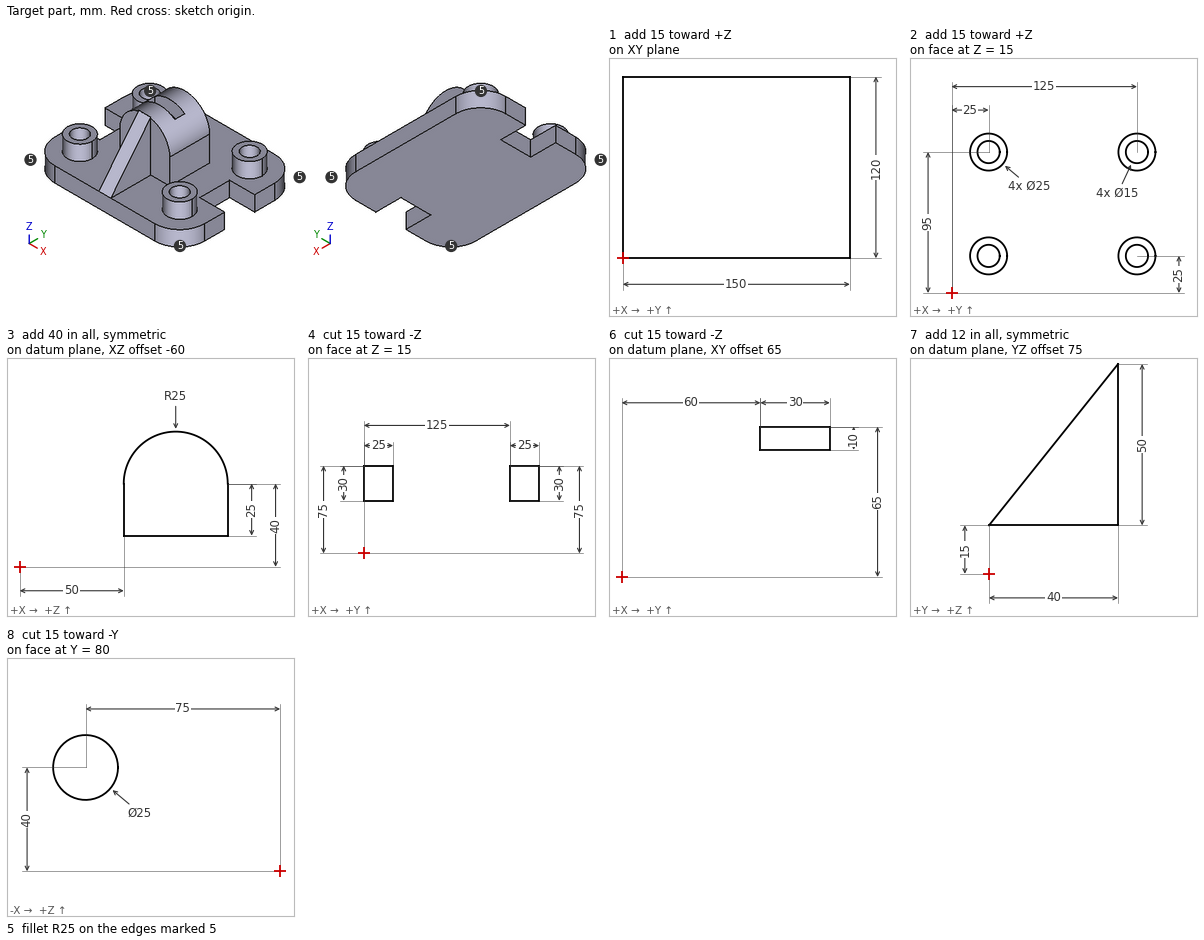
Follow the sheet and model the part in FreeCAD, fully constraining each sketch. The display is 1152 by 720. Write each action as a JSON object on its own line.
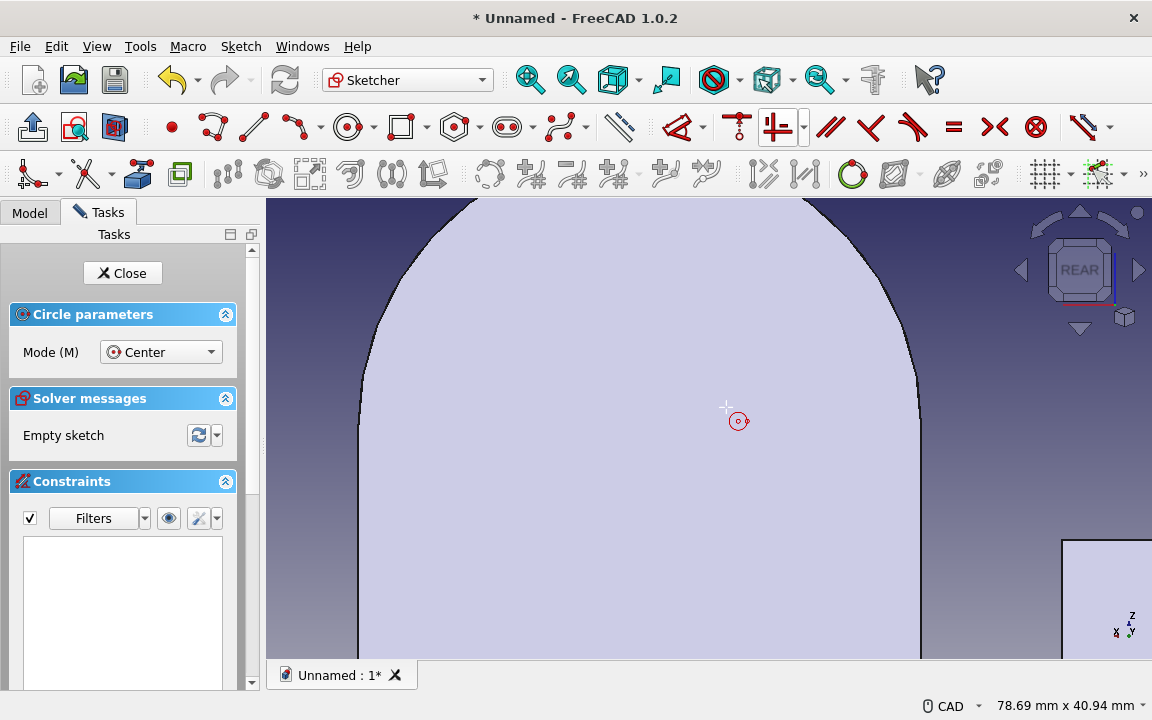
{"action": "left_click", "coordinate": [640, 427]}
{"action": "left_click", "coordinate": [739, 328]}
{"action": "key", "text": "Escape"}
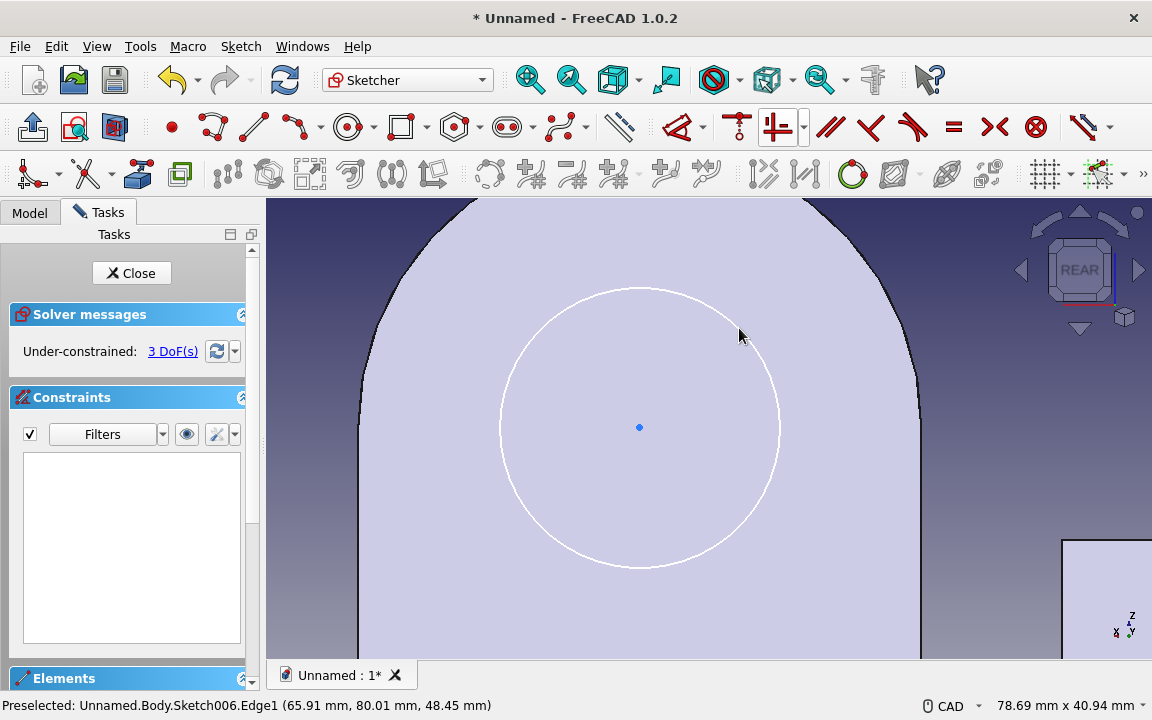
{"action": "left_click", "coordinate": [676, 128]}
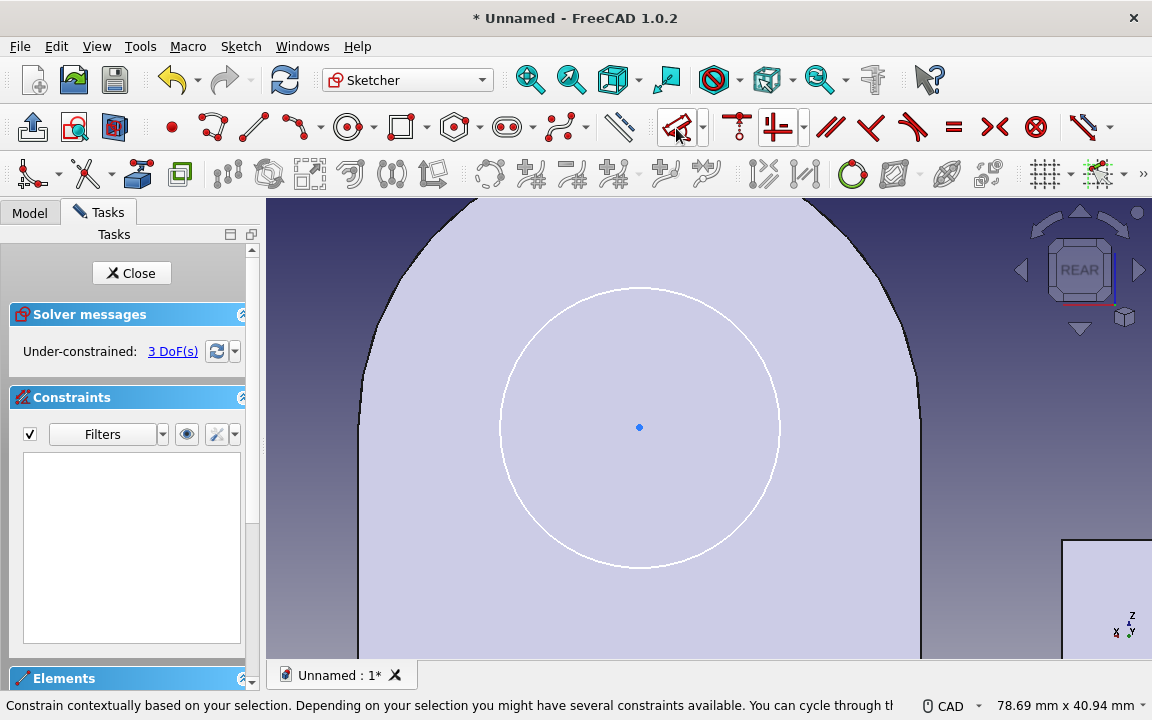
{"action": "left_click", "coordinate": [739, 329]}
{"action": "left_click", "coordinate": [762, 306]}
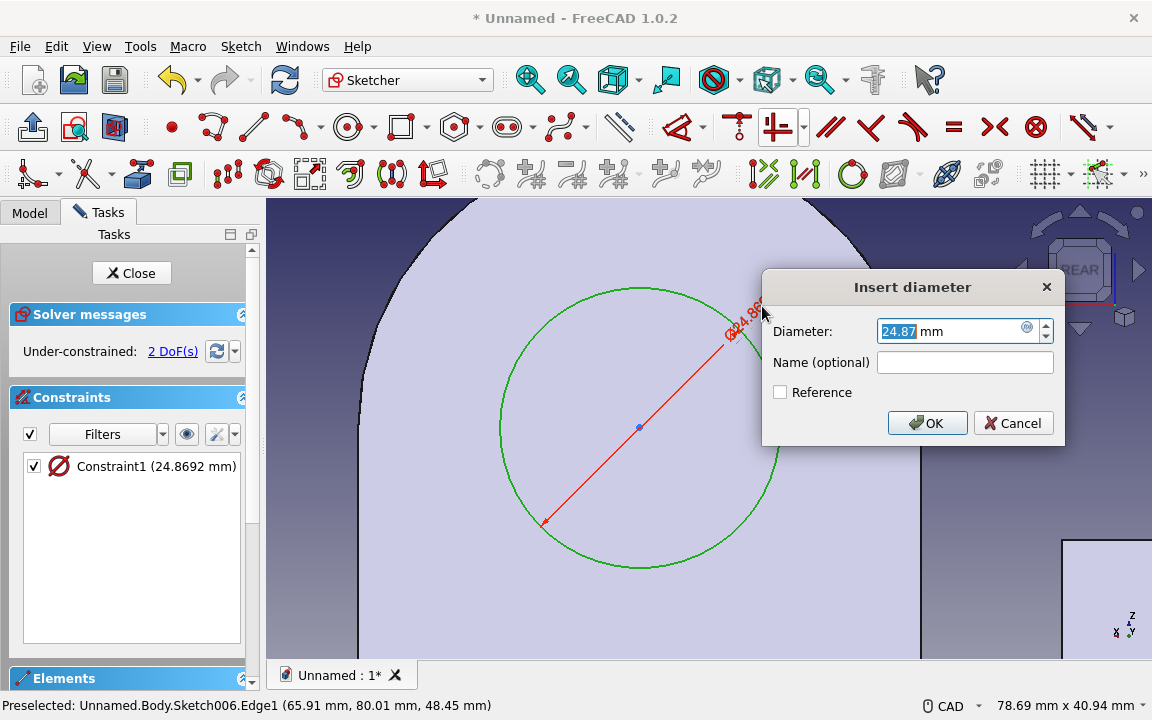
{"action": "type", "text": "25"}
{"action": "key", "text": "Return"}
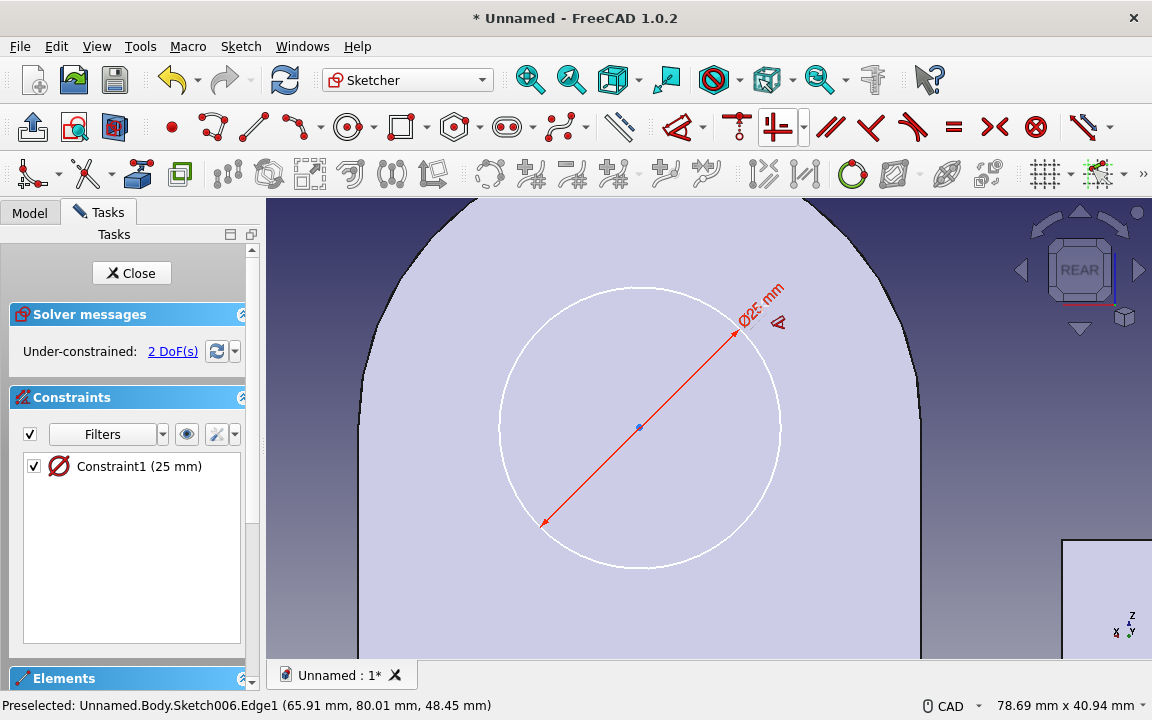
{"action": "left_click", "coordinate": [640, 428]}
{"action": "left_click", "coordinate": [814, 394]}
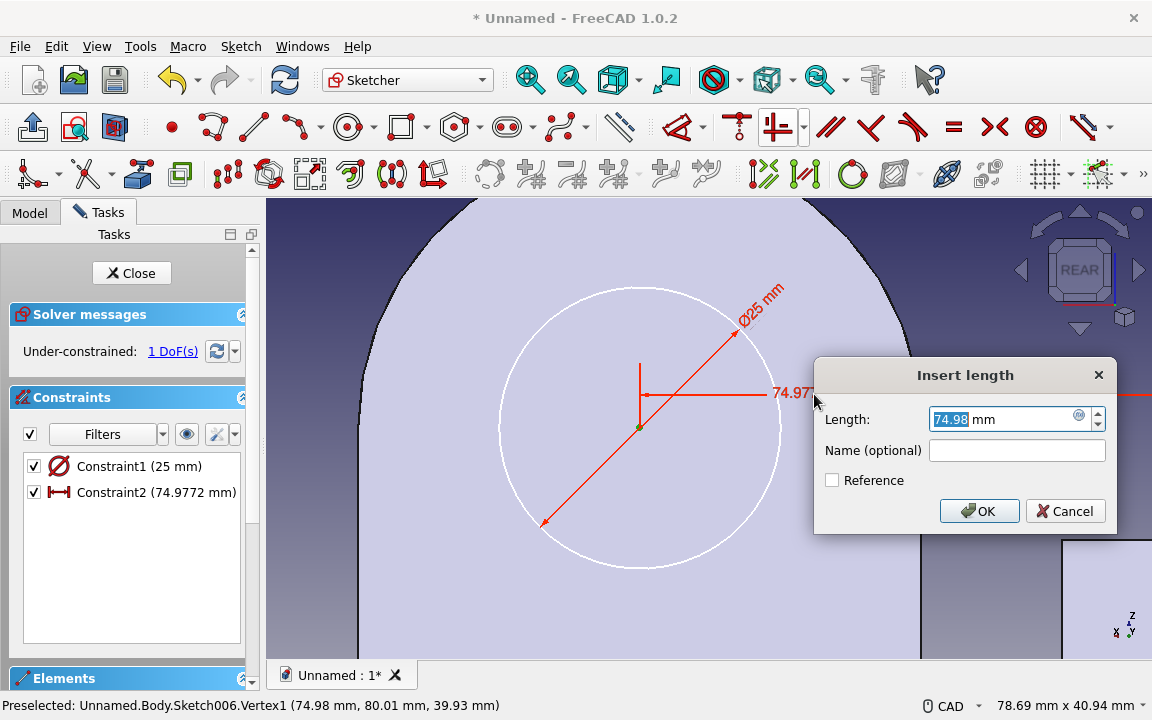
{"action": "type", "text": "75"}
{"action": "key", "text": "Return"}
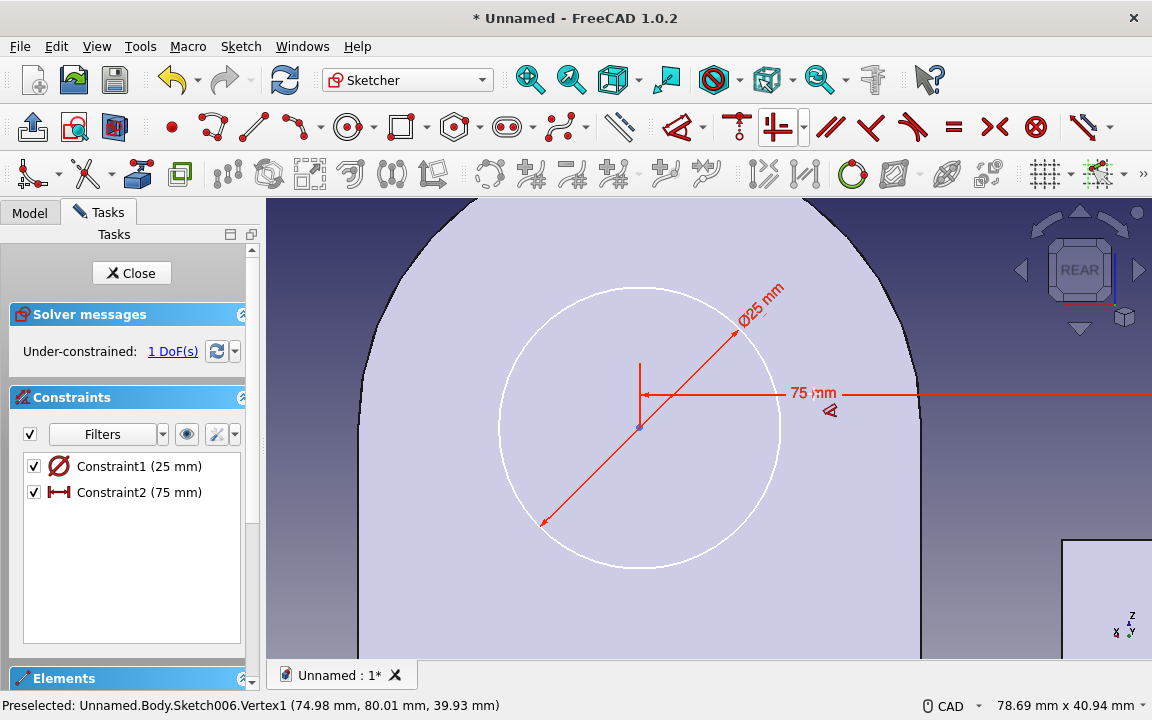
{"action": "left_click", "coordinate": [640, 428]}
{"action": "left_click", "coordinate": [606, 530]}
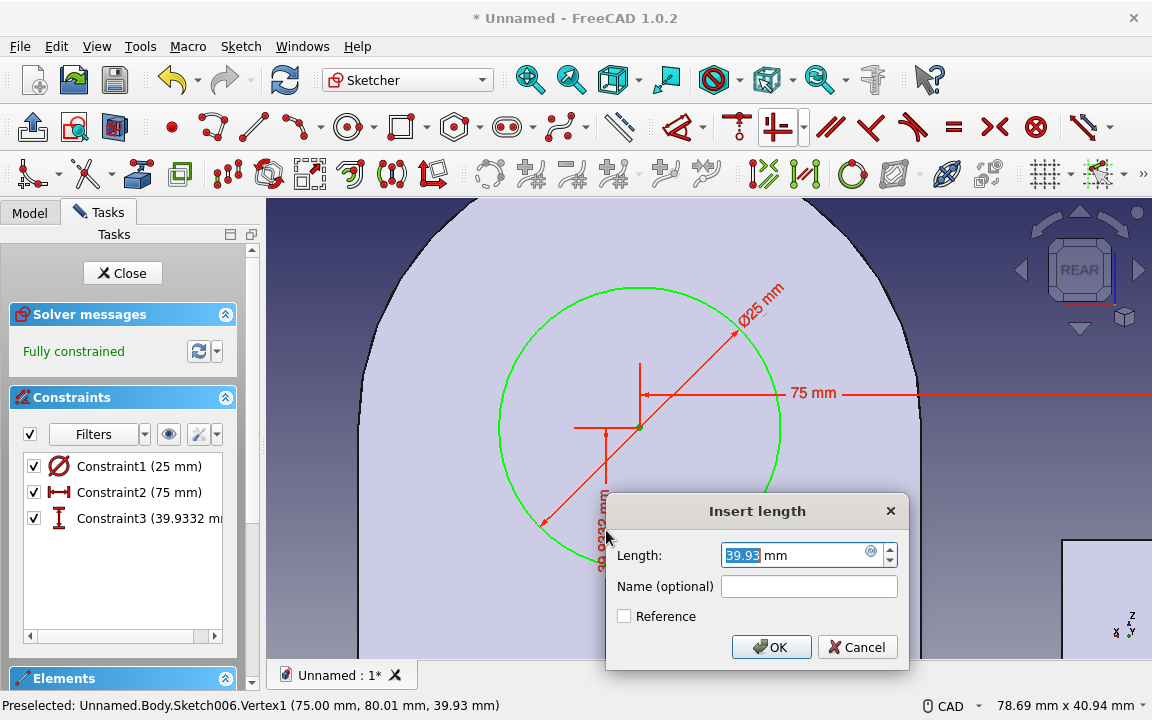
{"action": "type", "text": "40"}
{"action": "key", "text": "Return"}
{"action": "key", "text": "Escape"}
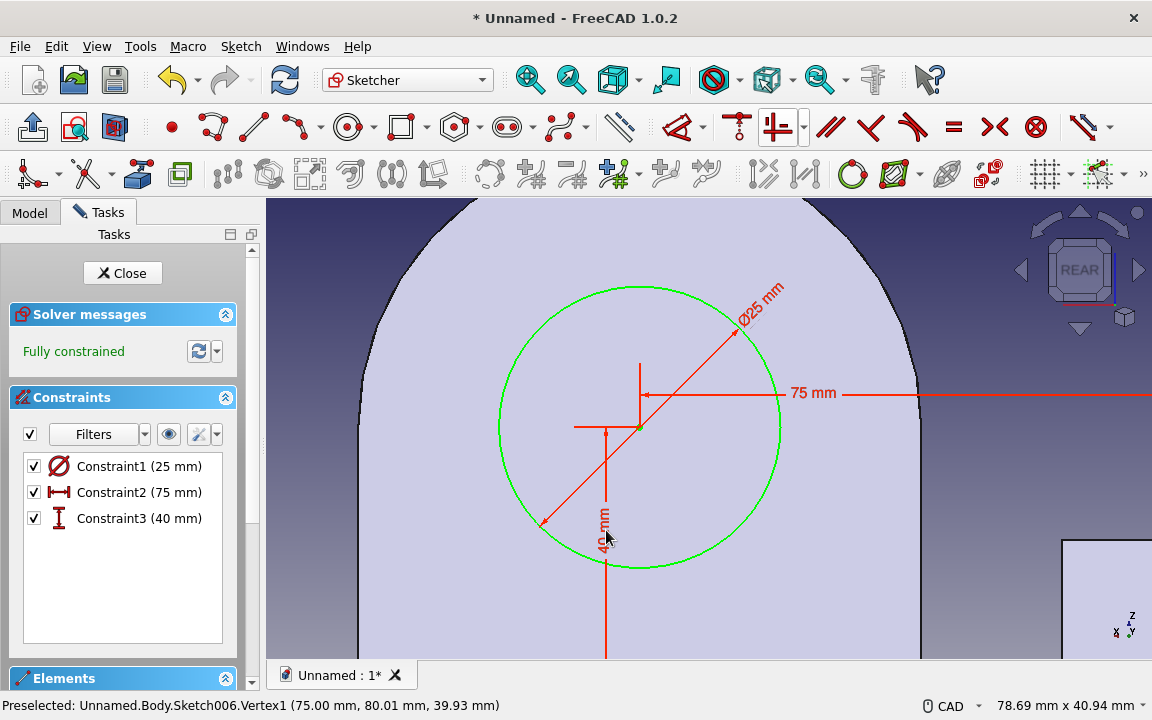
{"action": "left_click", "coordinate": [123, 273]}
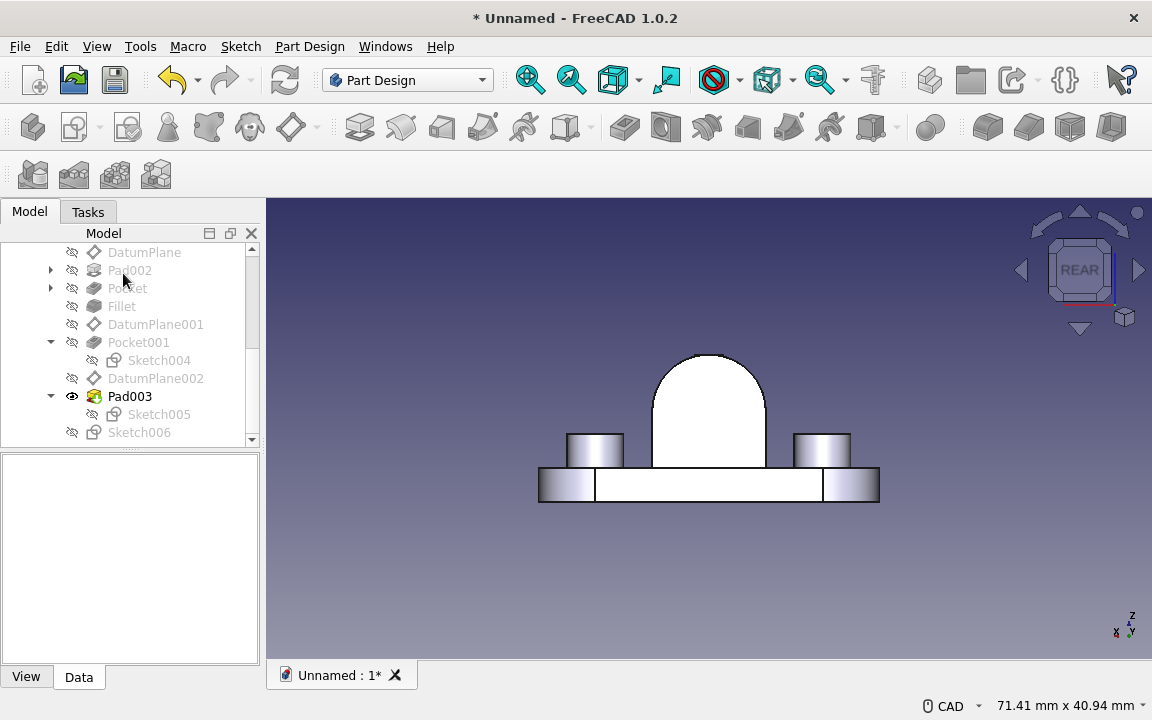
{"action": "left_click", "coordinate": [625, 128]}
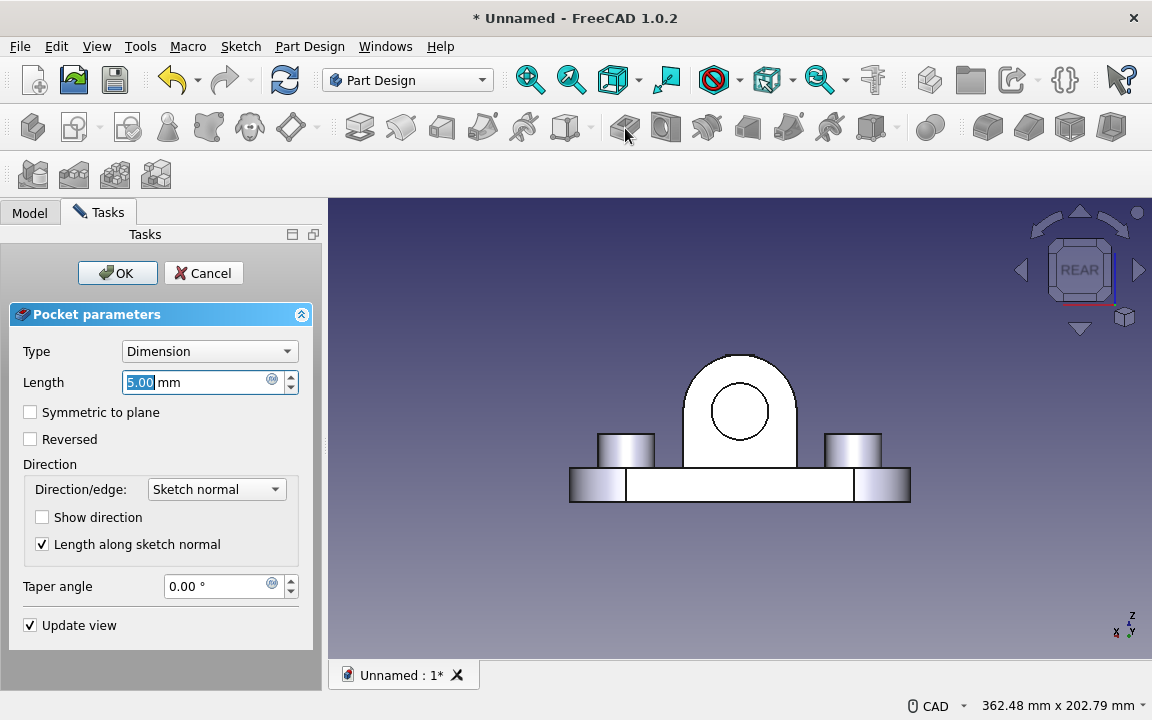
{"action": "type", "text": "15"}
{"action": "key", "text": "Tab"}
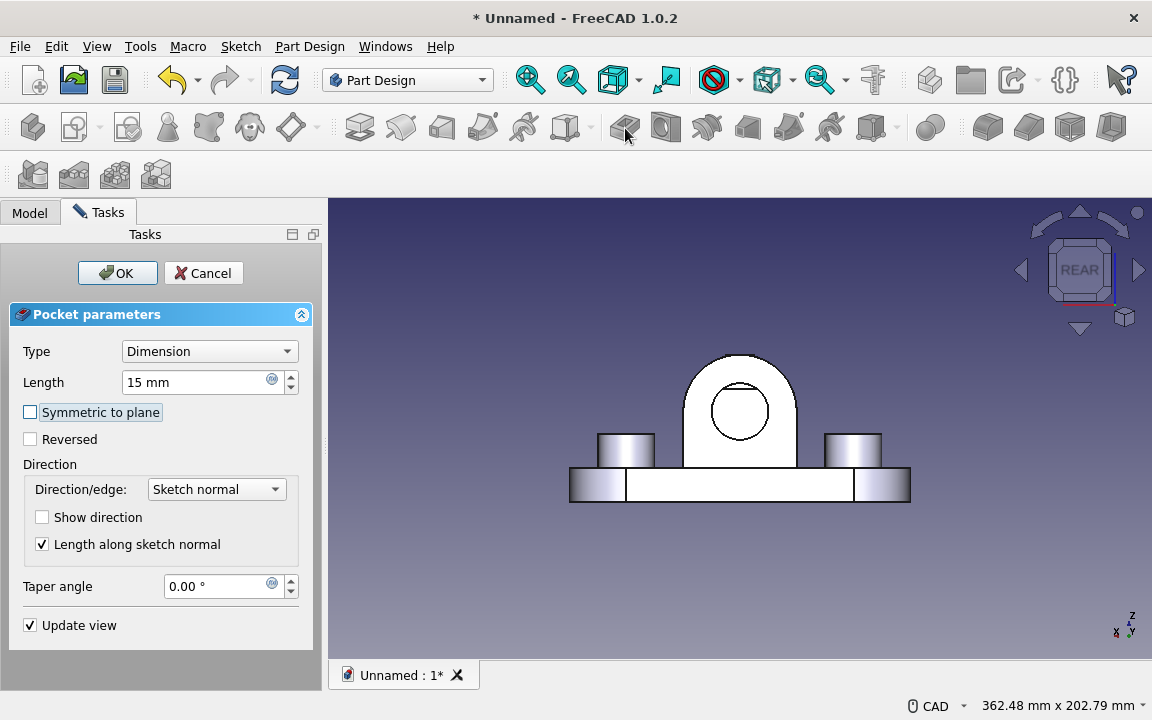
{"action": "left_click", "coordinate": [118, 273]}